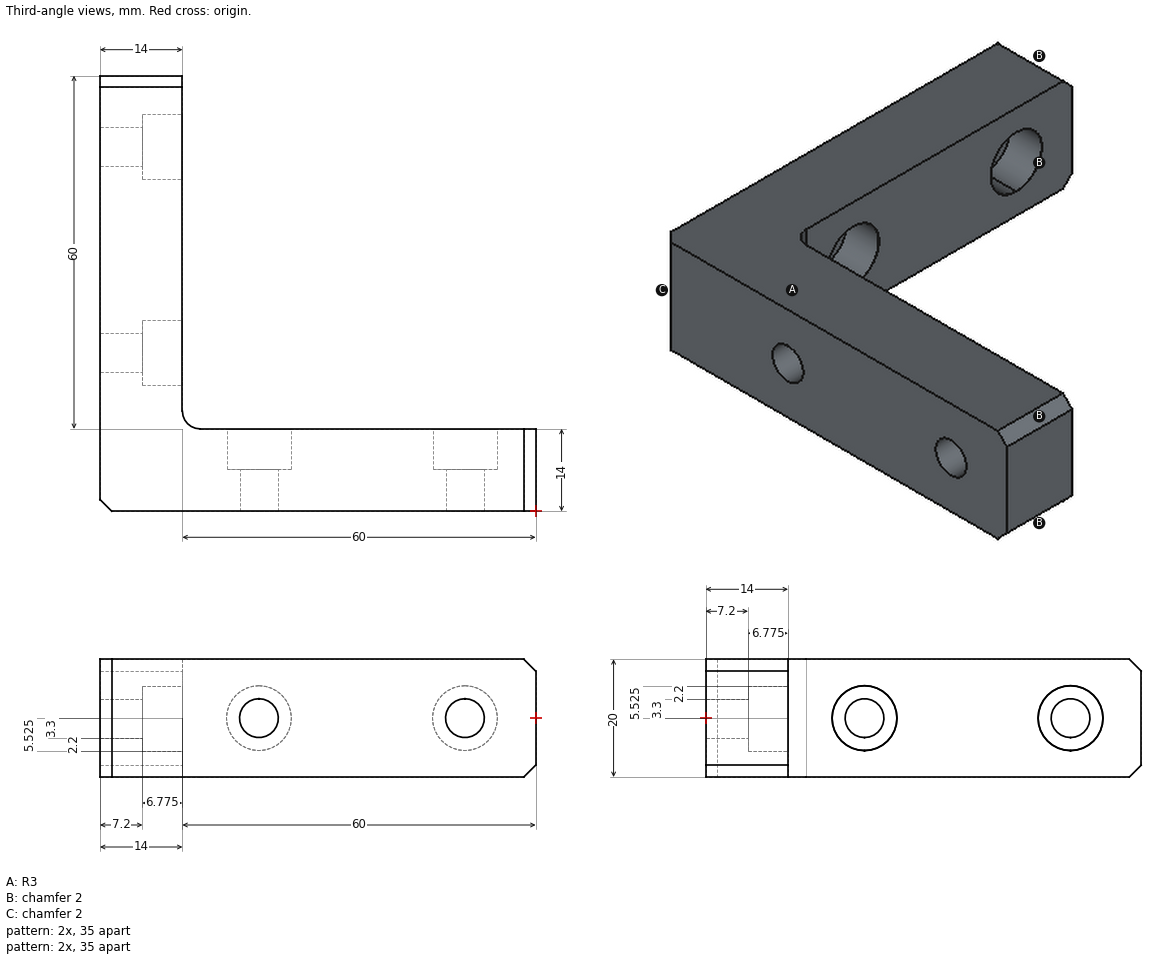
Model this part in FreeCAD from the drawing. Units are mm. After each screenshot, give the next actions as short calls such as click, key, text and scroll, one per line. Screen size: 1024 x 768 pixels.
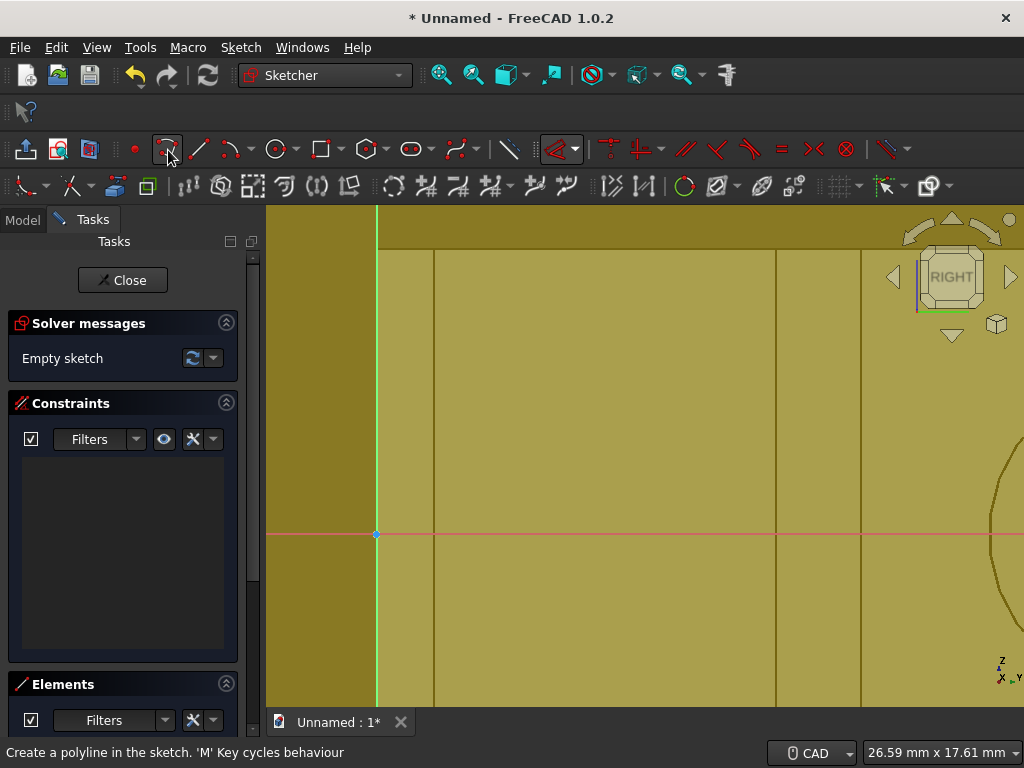
click(377, 534)
click(776, 525)
click(776, 377)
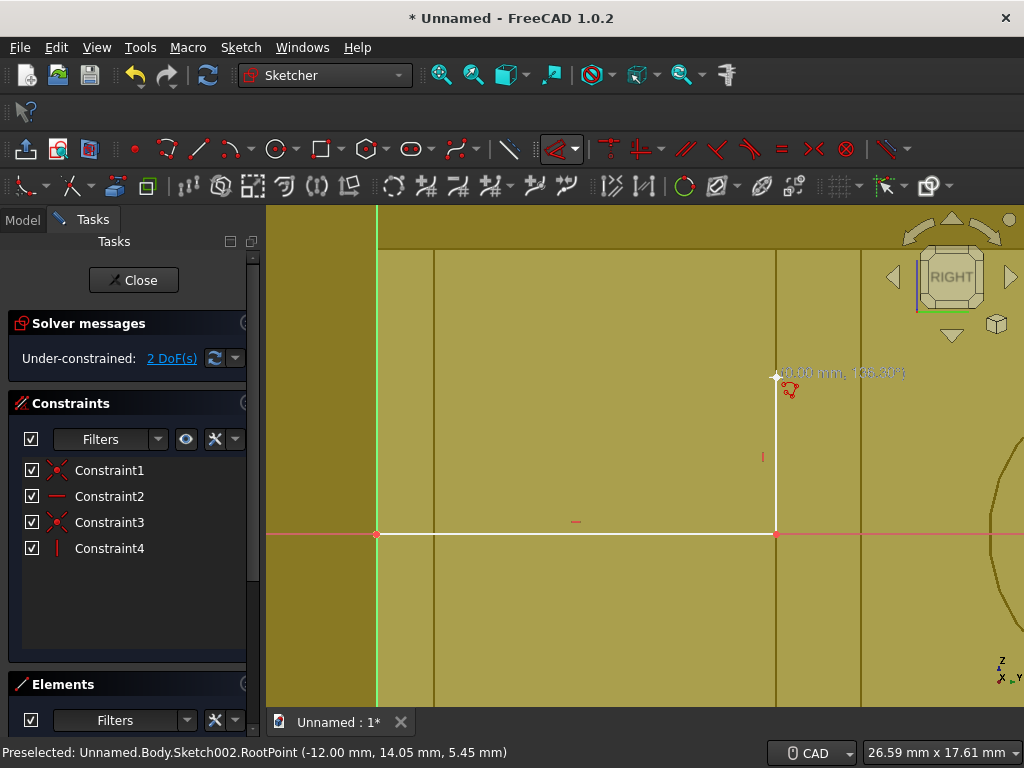
scroll(775, 378, up, 16)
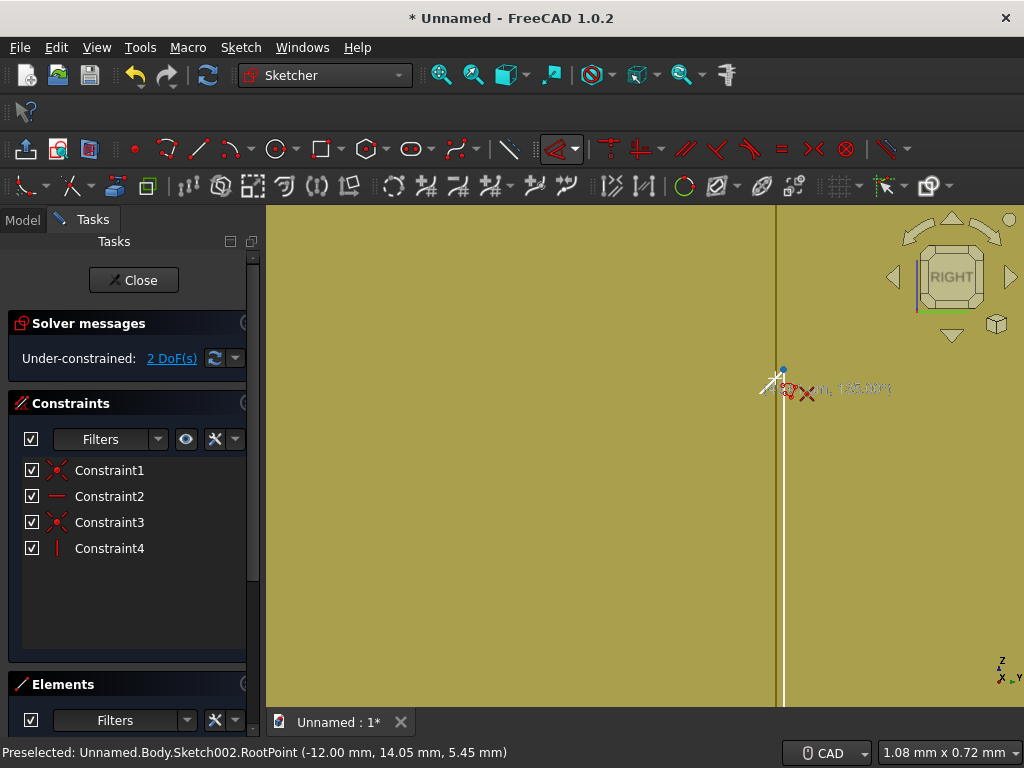
click(758, 361)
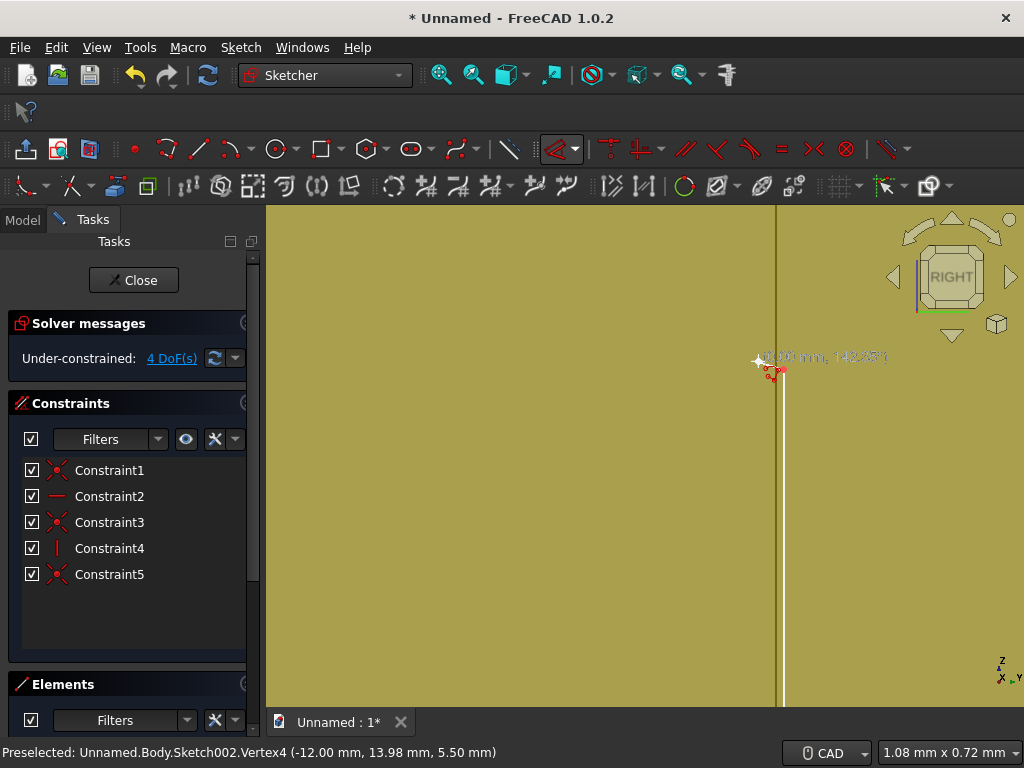
scroll(823, 361, down, 15)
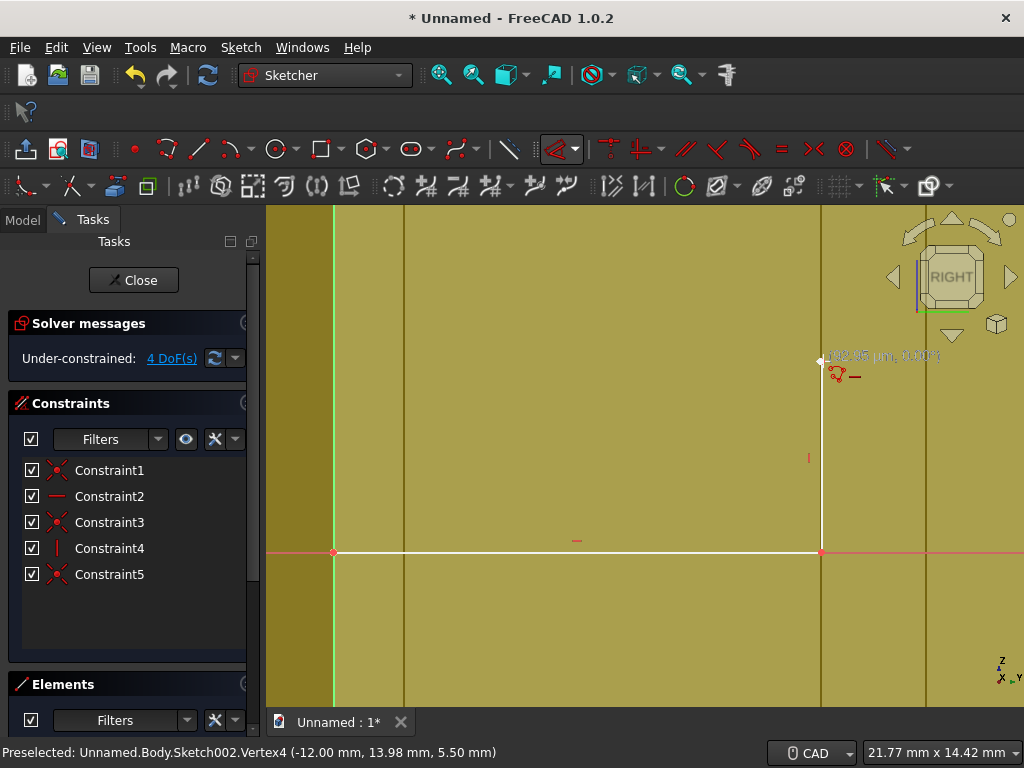
click(585, 361)
click(585, 438)
click(343, 438)
click(334, 553)
key(Escape)
key(Escape)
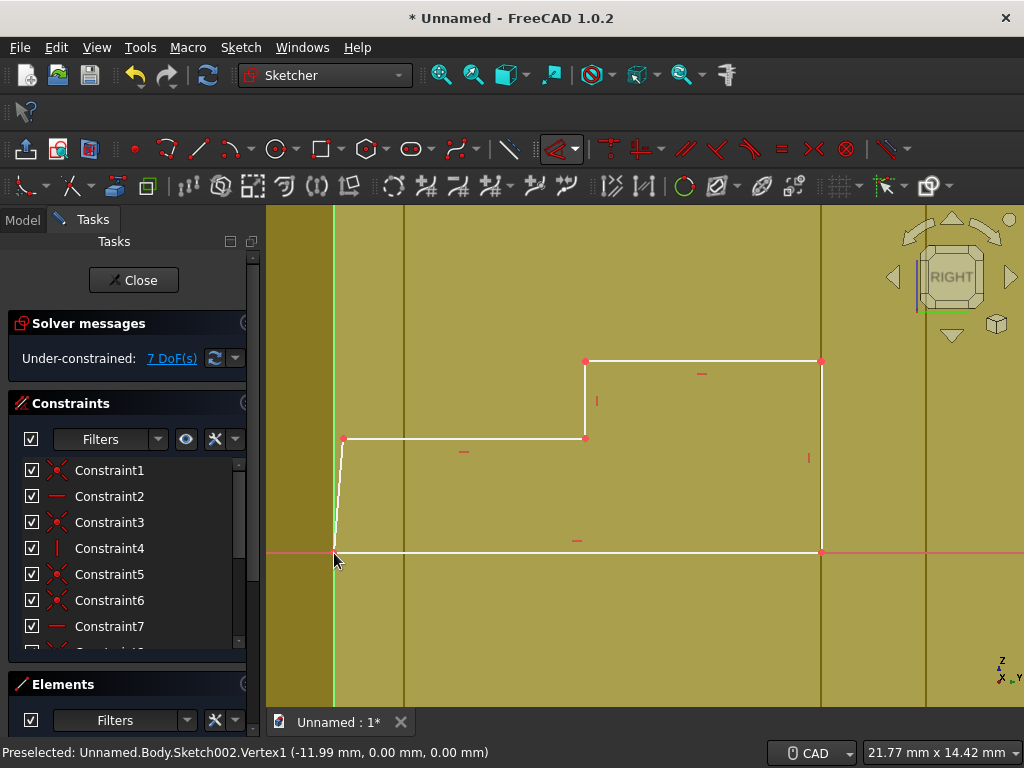
click(337, 519)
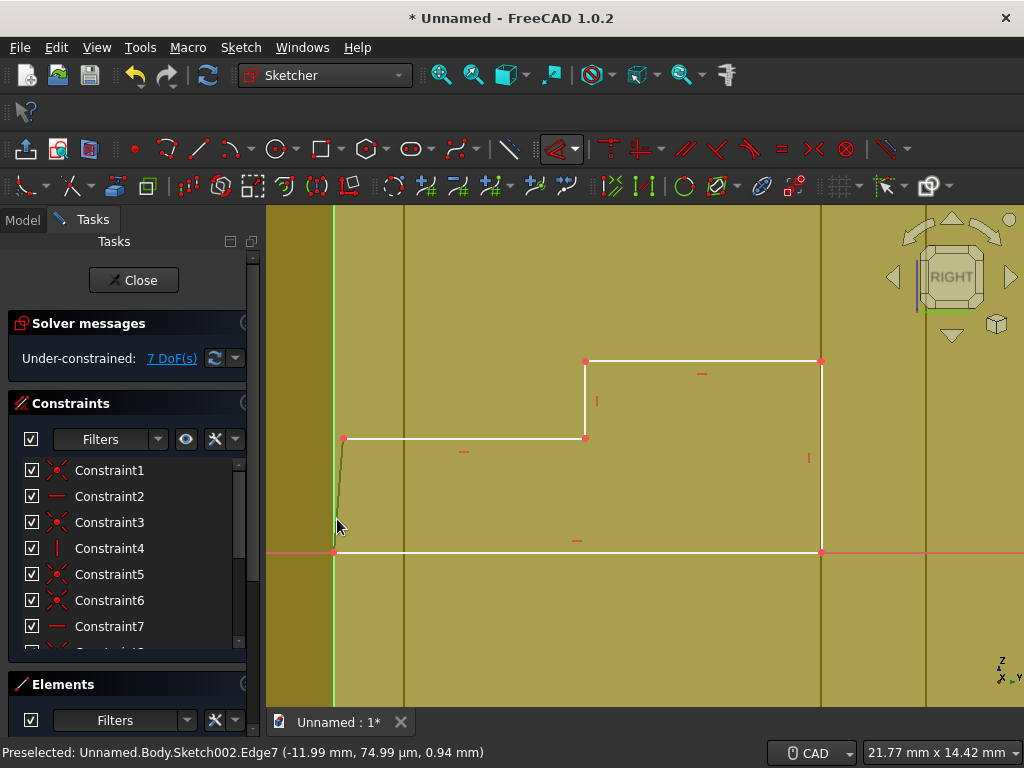
key(v)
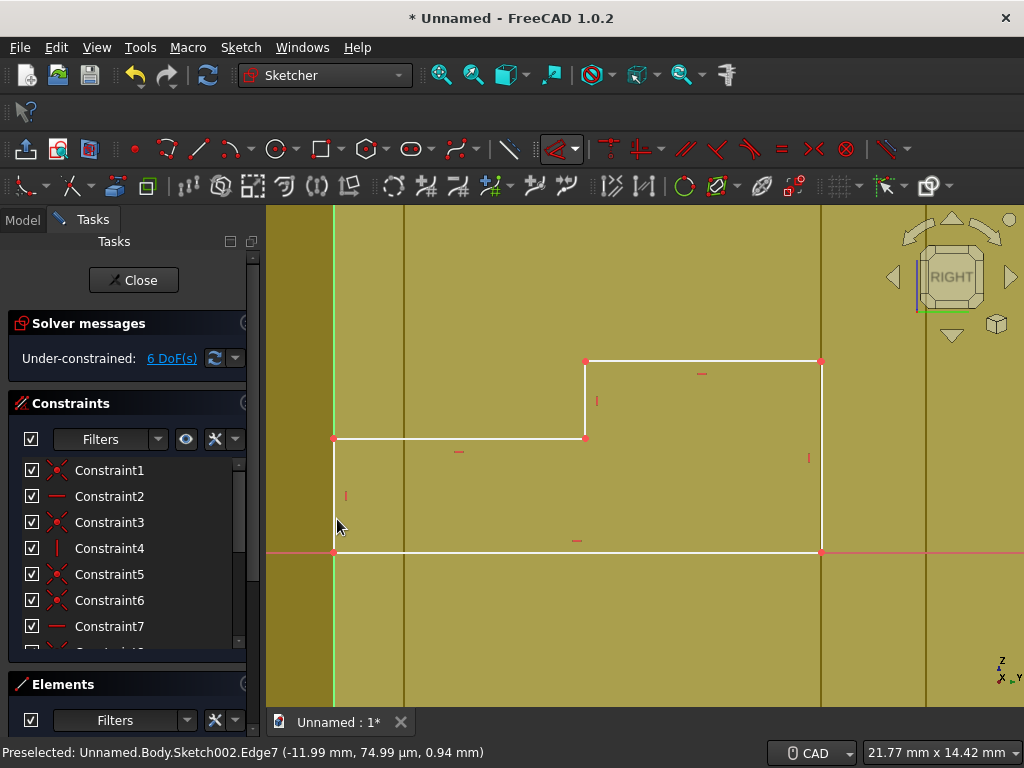
click(480, 553)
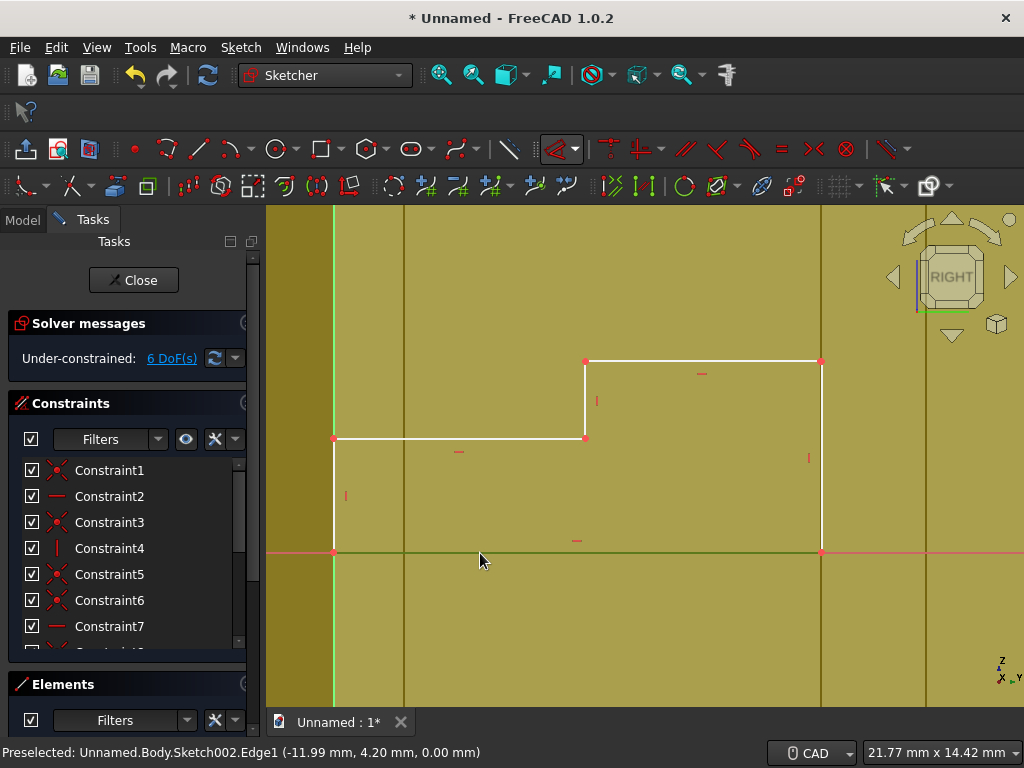
click(578, 150)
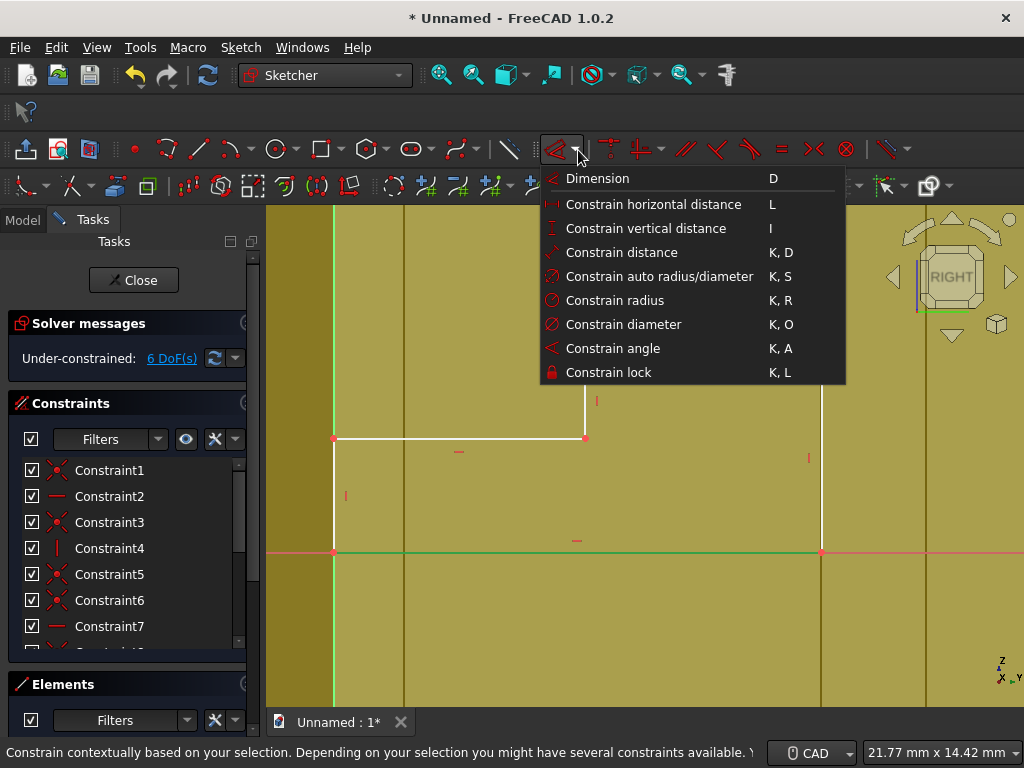
click(693, 204)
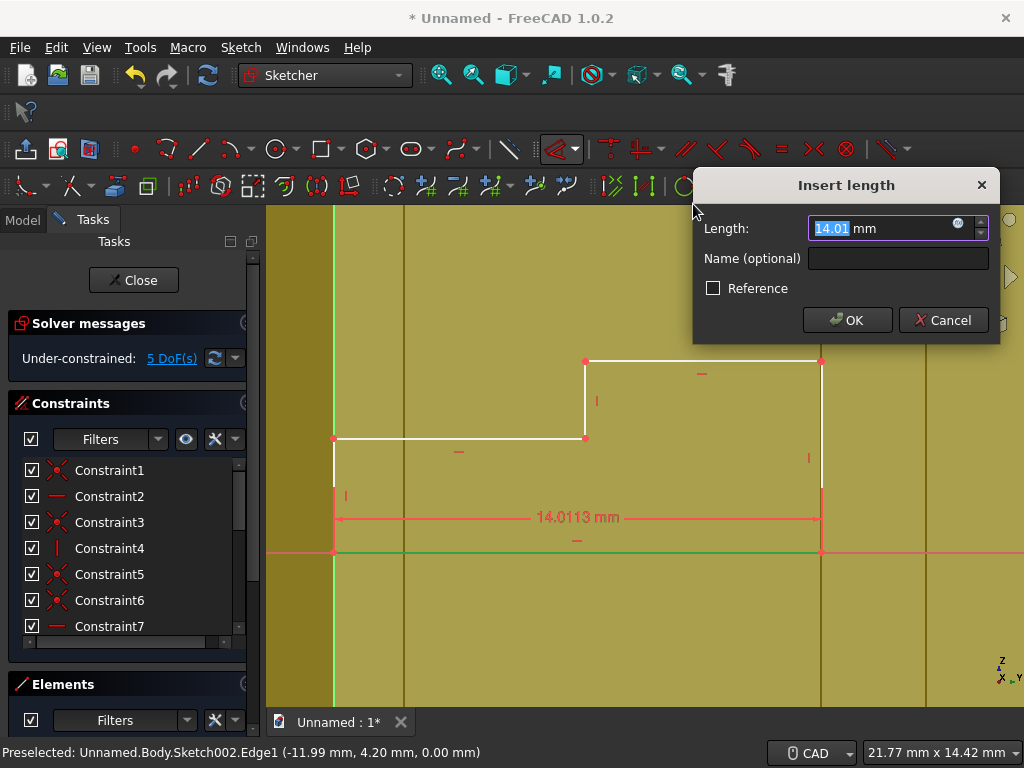
text(14)
key(Return)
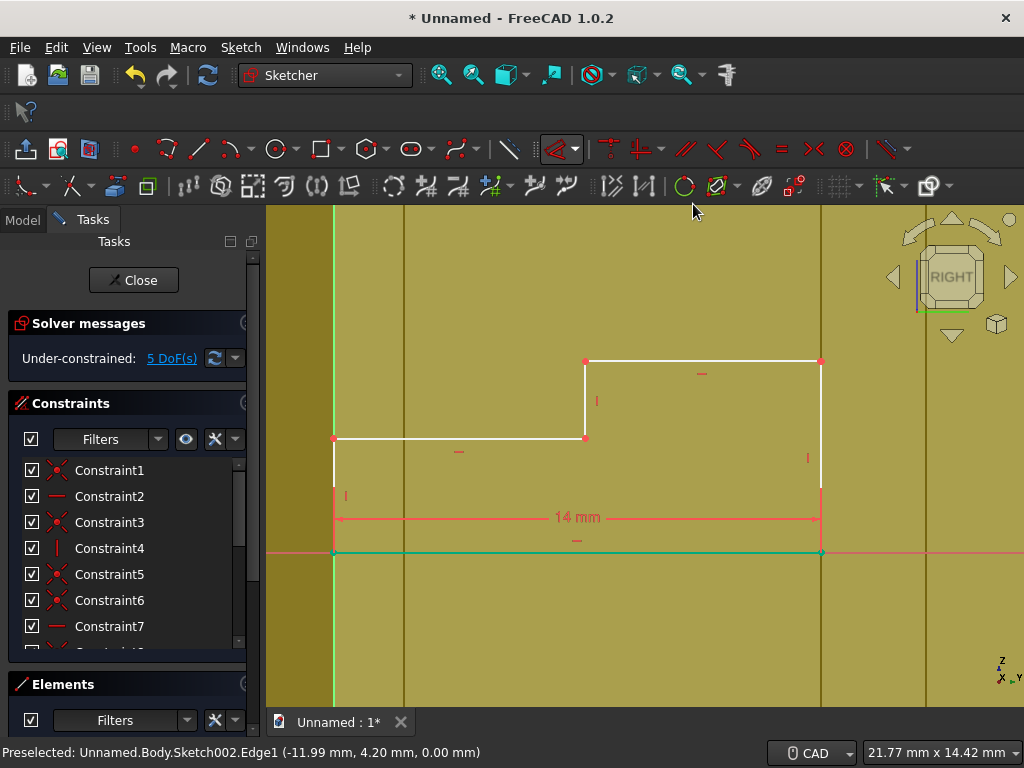
click(585, 385)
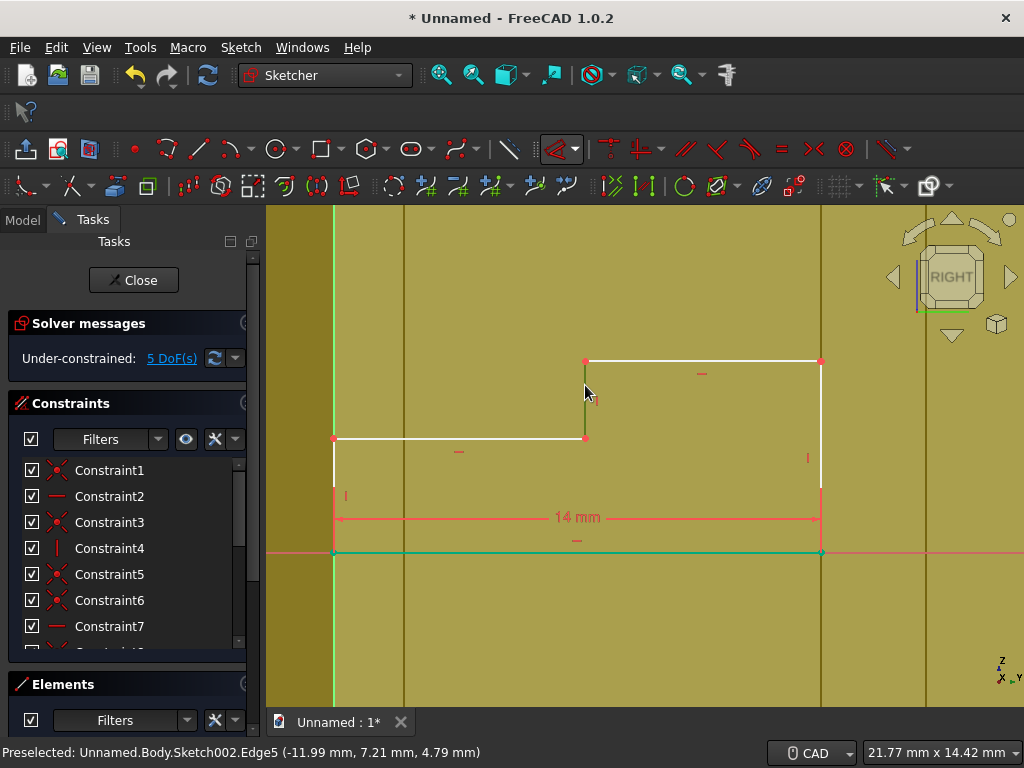
click(578, 150)